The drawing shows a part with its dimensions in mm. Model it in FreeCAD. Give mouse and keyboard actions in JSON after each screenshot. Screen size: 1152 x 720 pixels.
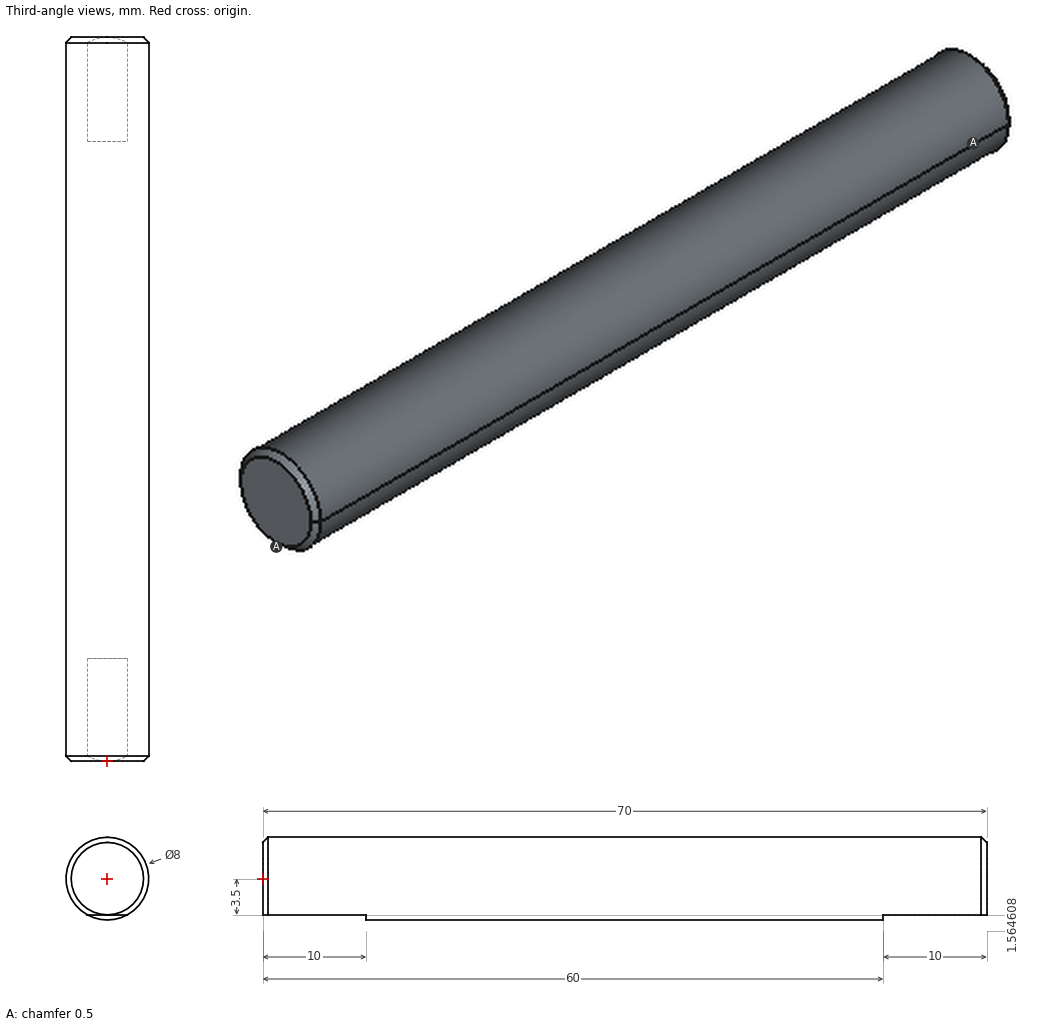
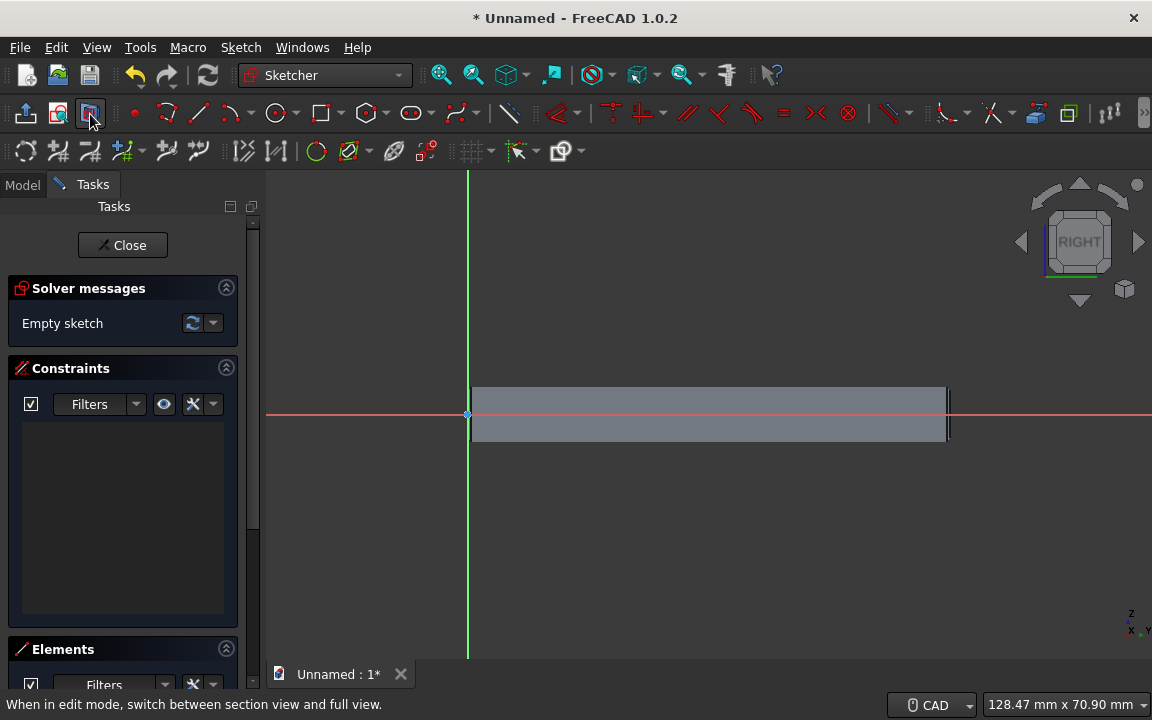
{"action": "key", "text": "g r"}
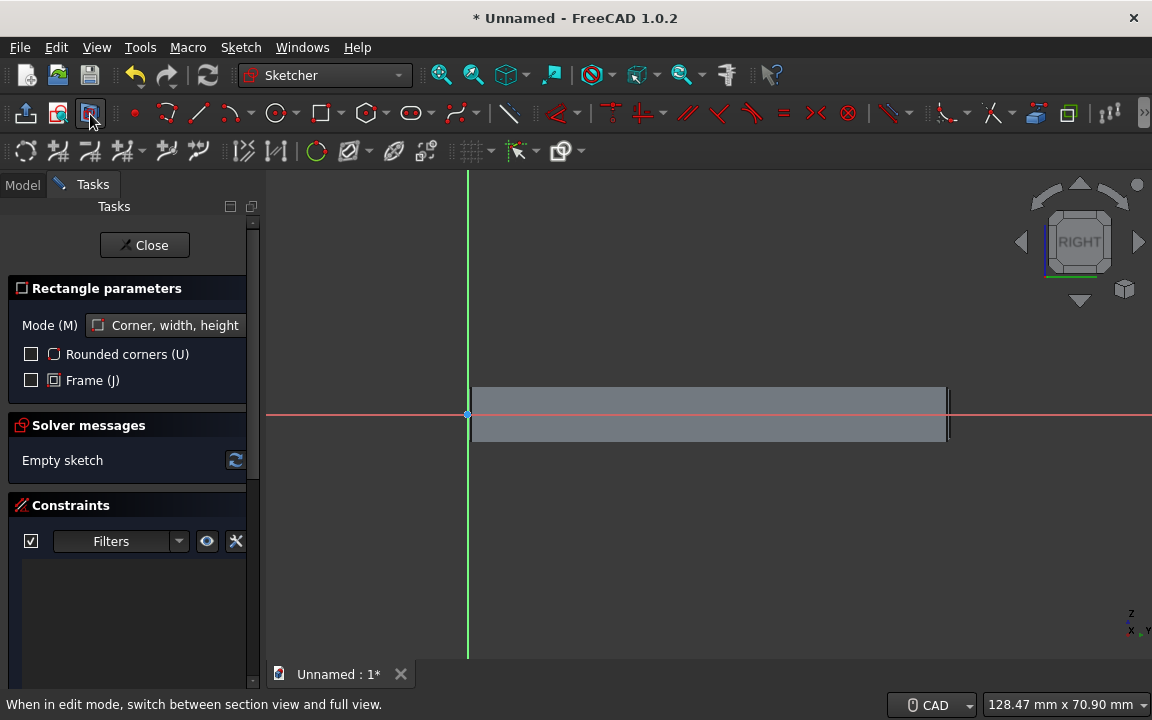
{"action": "scroll", "coordinate": [881, 439], "scroll_direction": "up", "scroll_amount": 2}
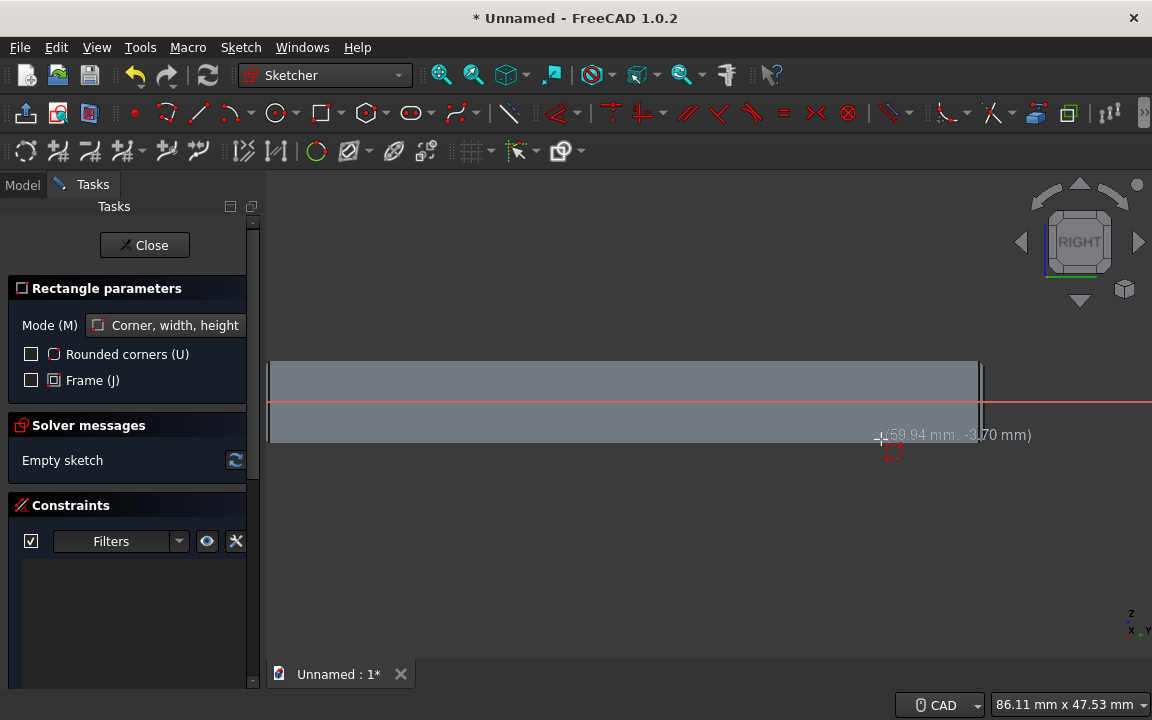
{"action": "left_click", "coordinate": [881, 438]}
{"action": "mouse_move", "coordinate": [984, 454]}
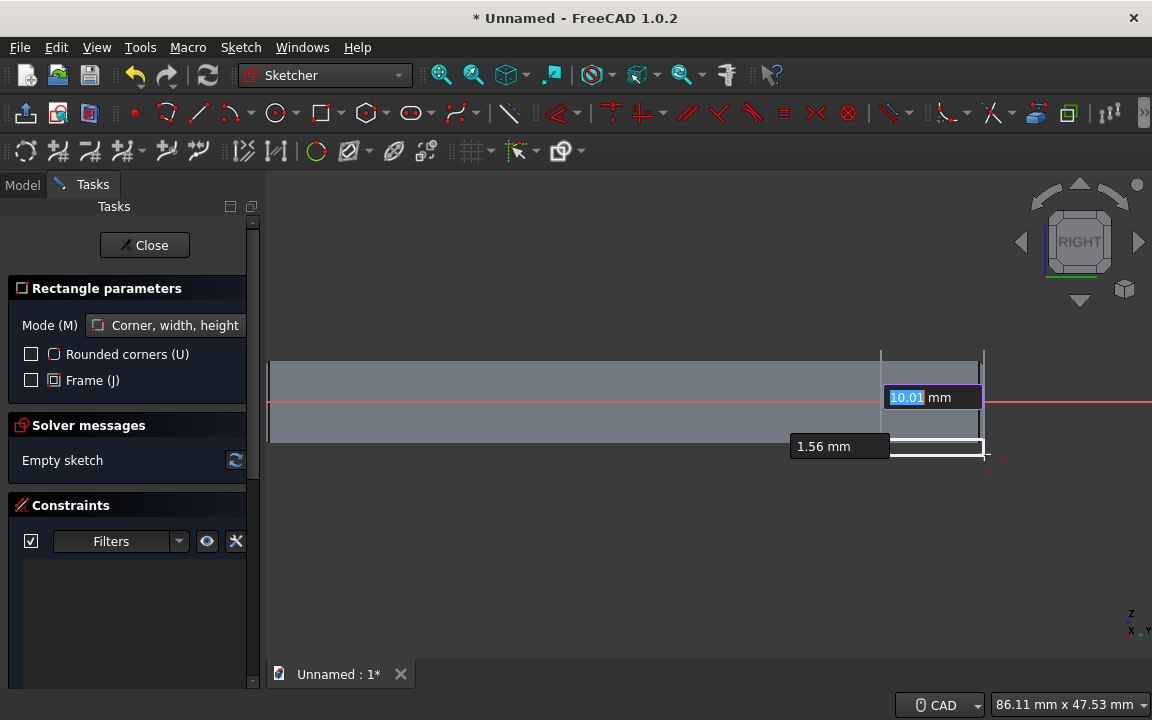
{"action": "type", "text": "10"}
{"action": "key", "text": "Tab"}
{"action": "type", "text": "1.564608"}
{"action": "key", "text": "Return"}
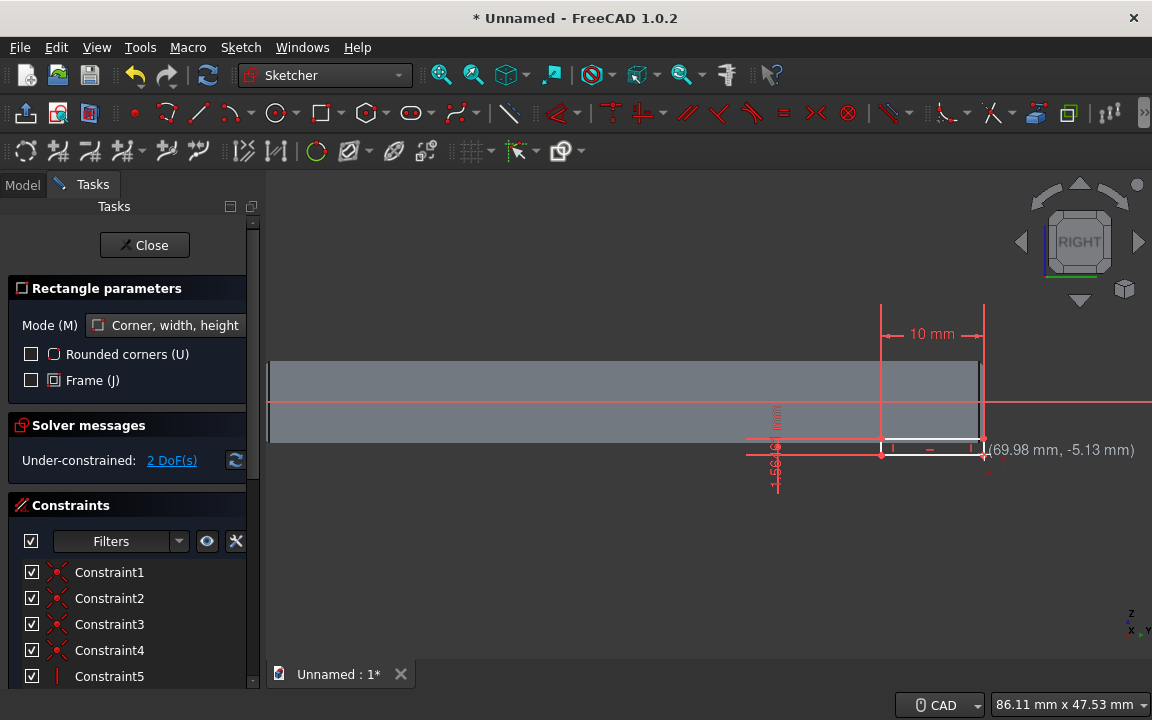
{"action": "scroll", "coordinate": [674, 387], "scroll_direction": "down", "scroll_amount": 2}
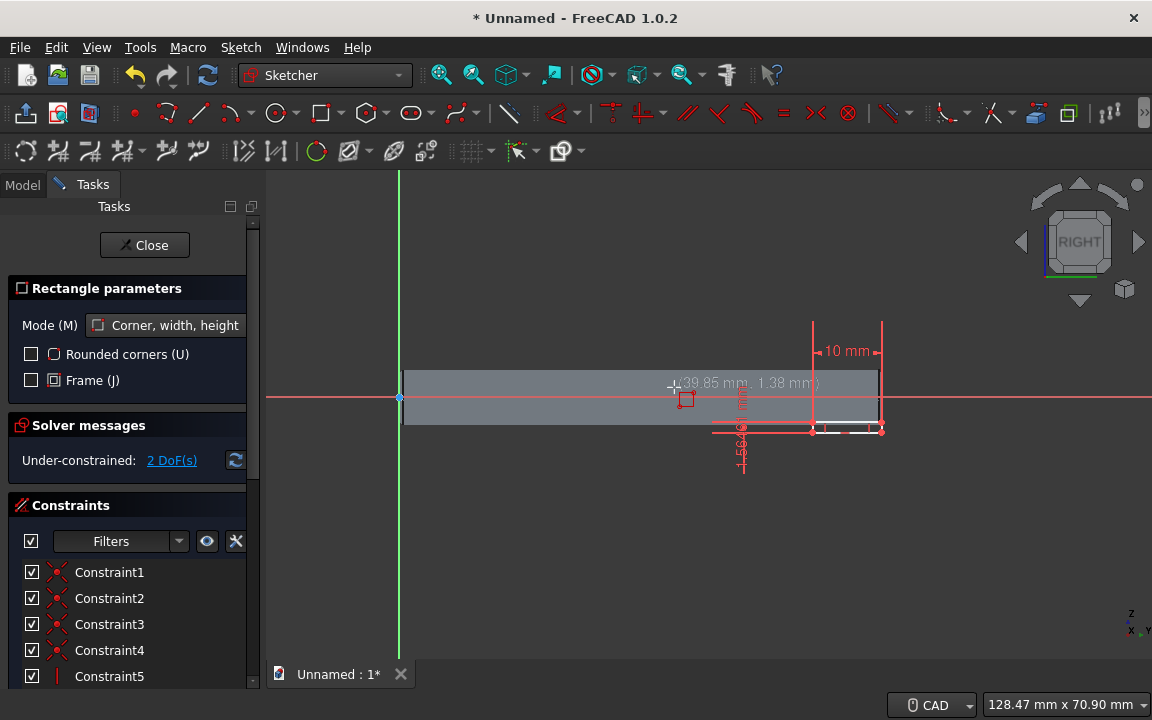
{"action": "scroll", "coordinate": [399, 421], "scroll_direction": "up", "scroll_amount": 2}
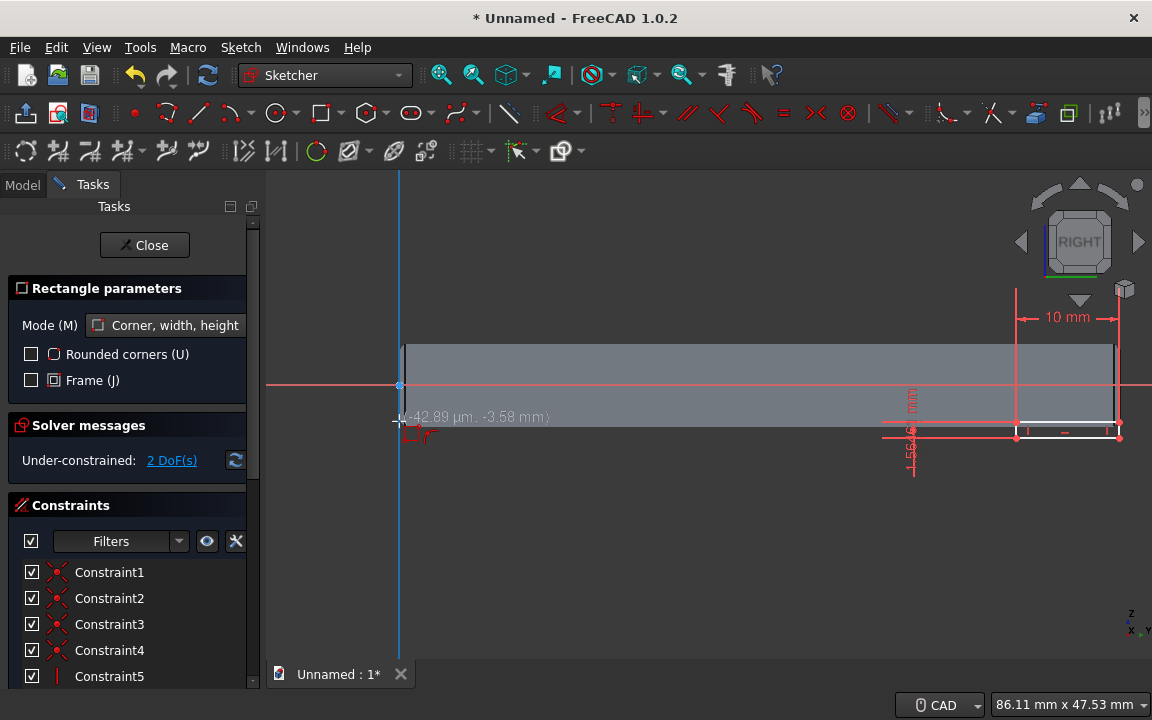
{"action": "left_click", "coordinate": [399, 421]}
{"action": "mouse_move", "coordinate": [502, 438]}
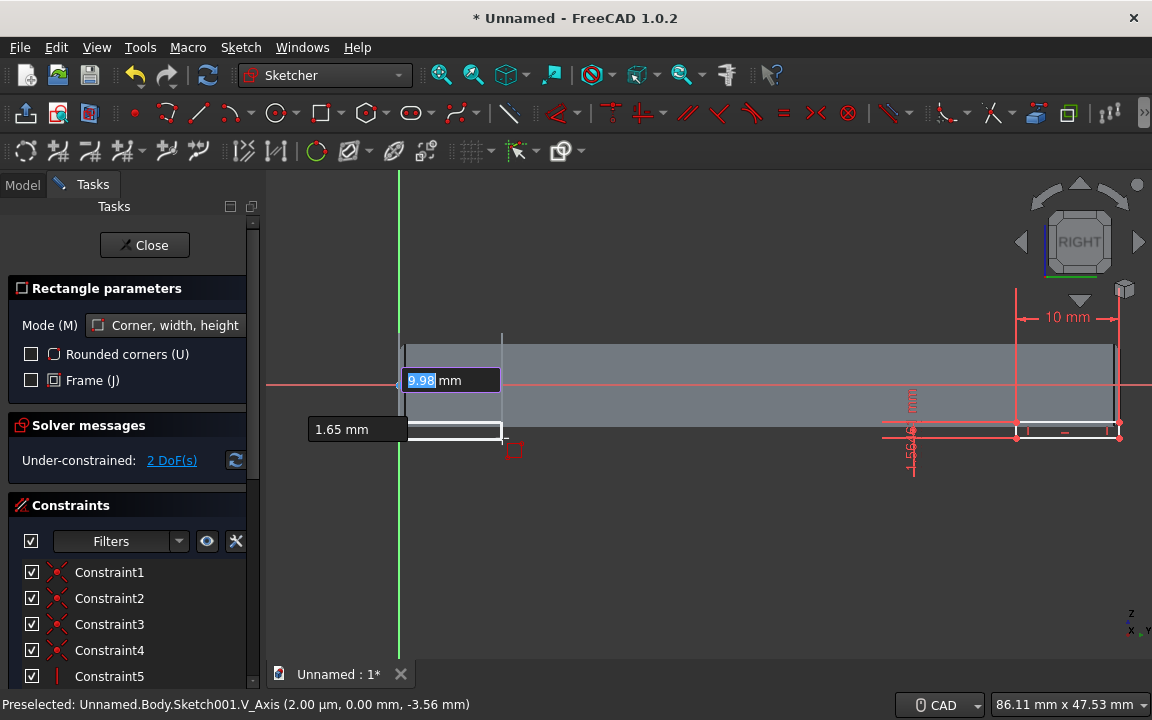
{"action": "type", "text": "10"}
{"action": "key", "text": "Tab"}
{"action": "type", "text": "1.564608"}
{"action": "key", "text": "Return"}
{"action": "key", "text": "Escape"}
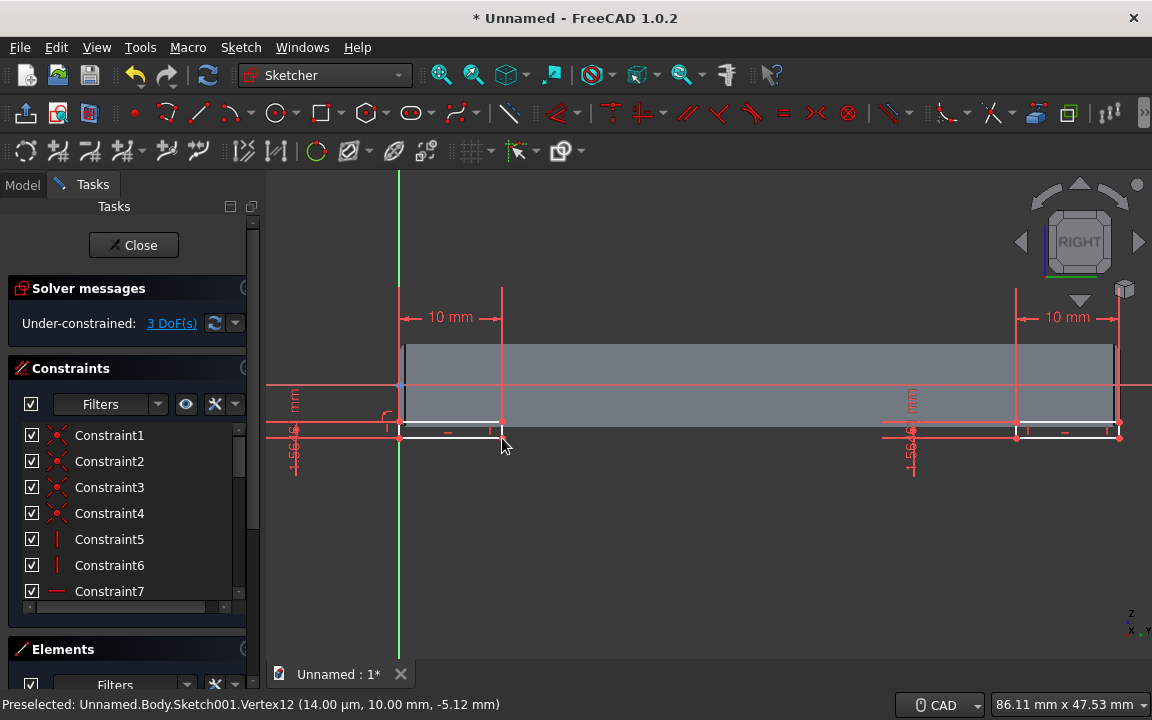
{"action": "left_click", "coordinate": [556, 114]}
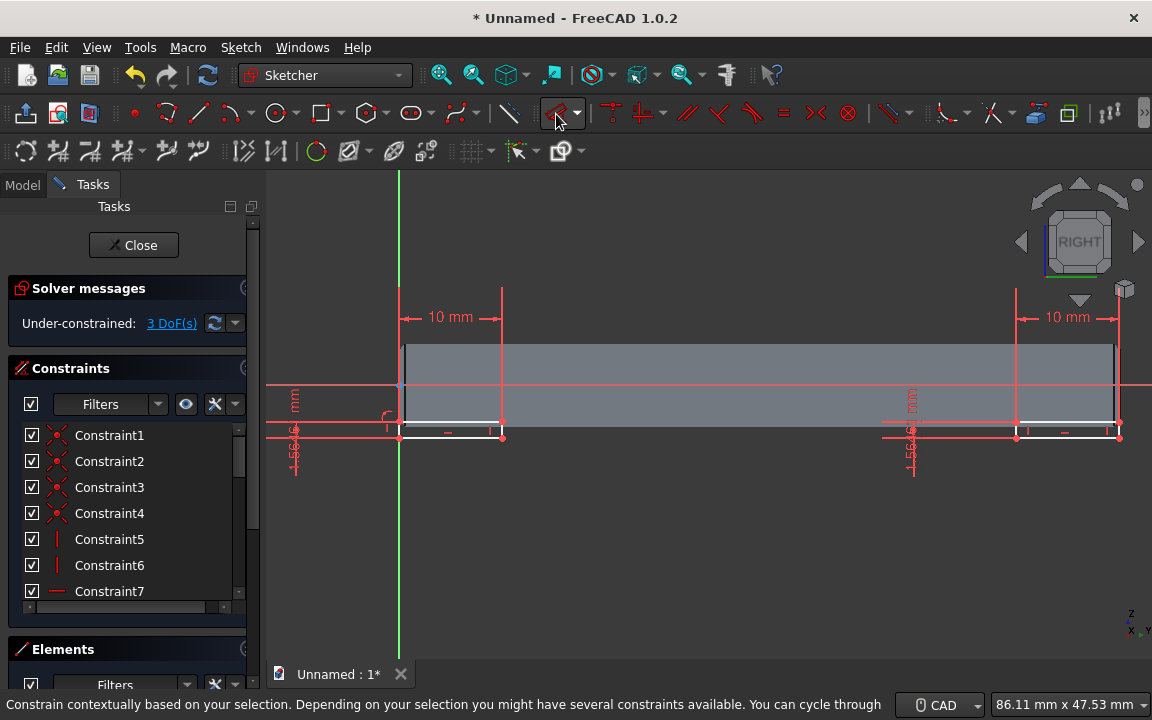
{"action": "scroll", "coordinate": [399, 421], "scroll_direction": "down", "scroll_amount": 2}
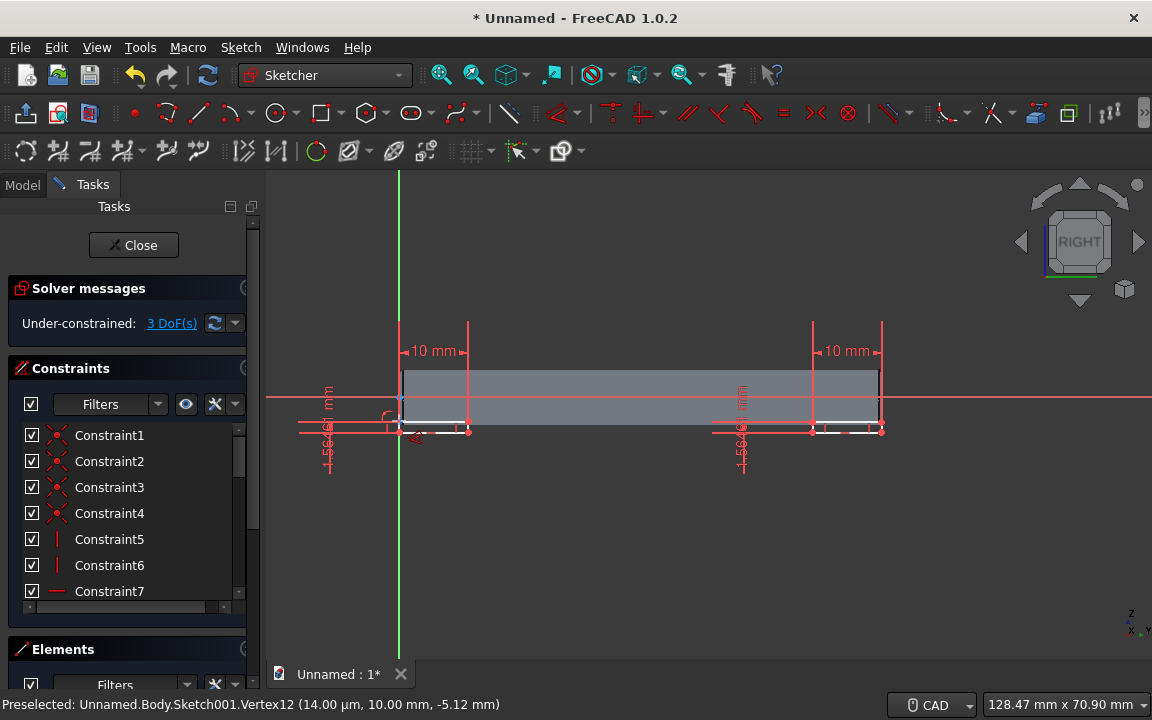
{"action": "left_click", "coordinate": [813, 422]}
{"action": "left_click", "coordinate": [606, 363]}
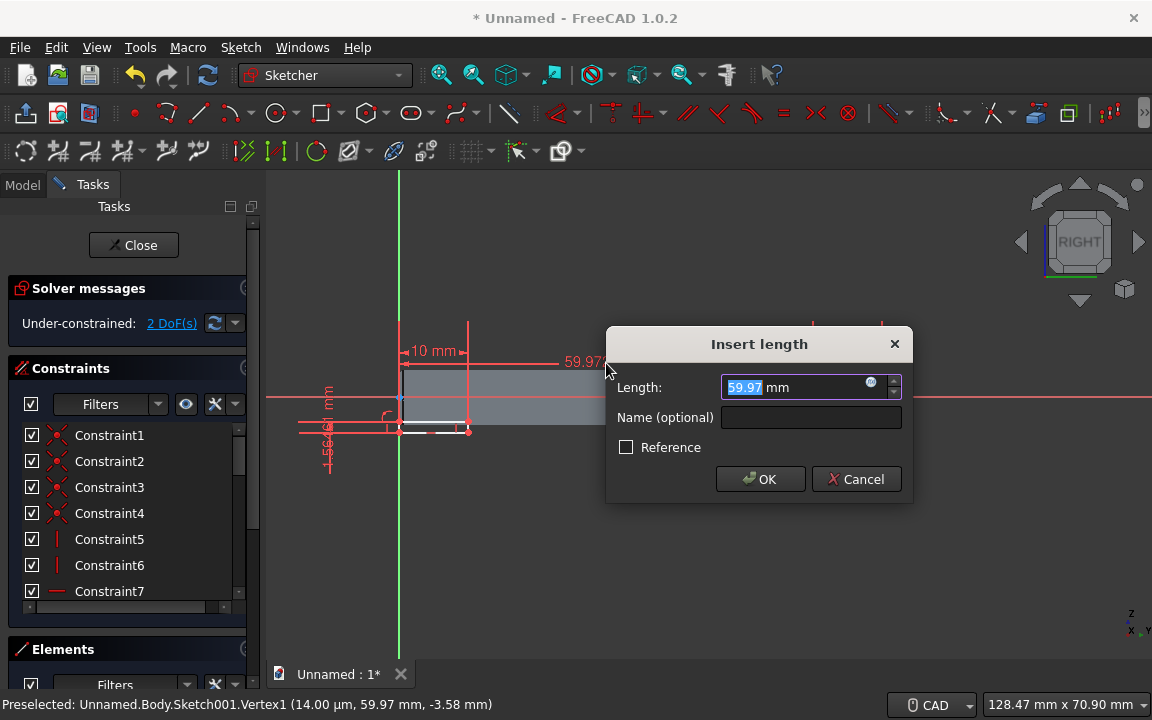
{"action": "type", "text": "60"}
{"action": "key", "text": "Return"}